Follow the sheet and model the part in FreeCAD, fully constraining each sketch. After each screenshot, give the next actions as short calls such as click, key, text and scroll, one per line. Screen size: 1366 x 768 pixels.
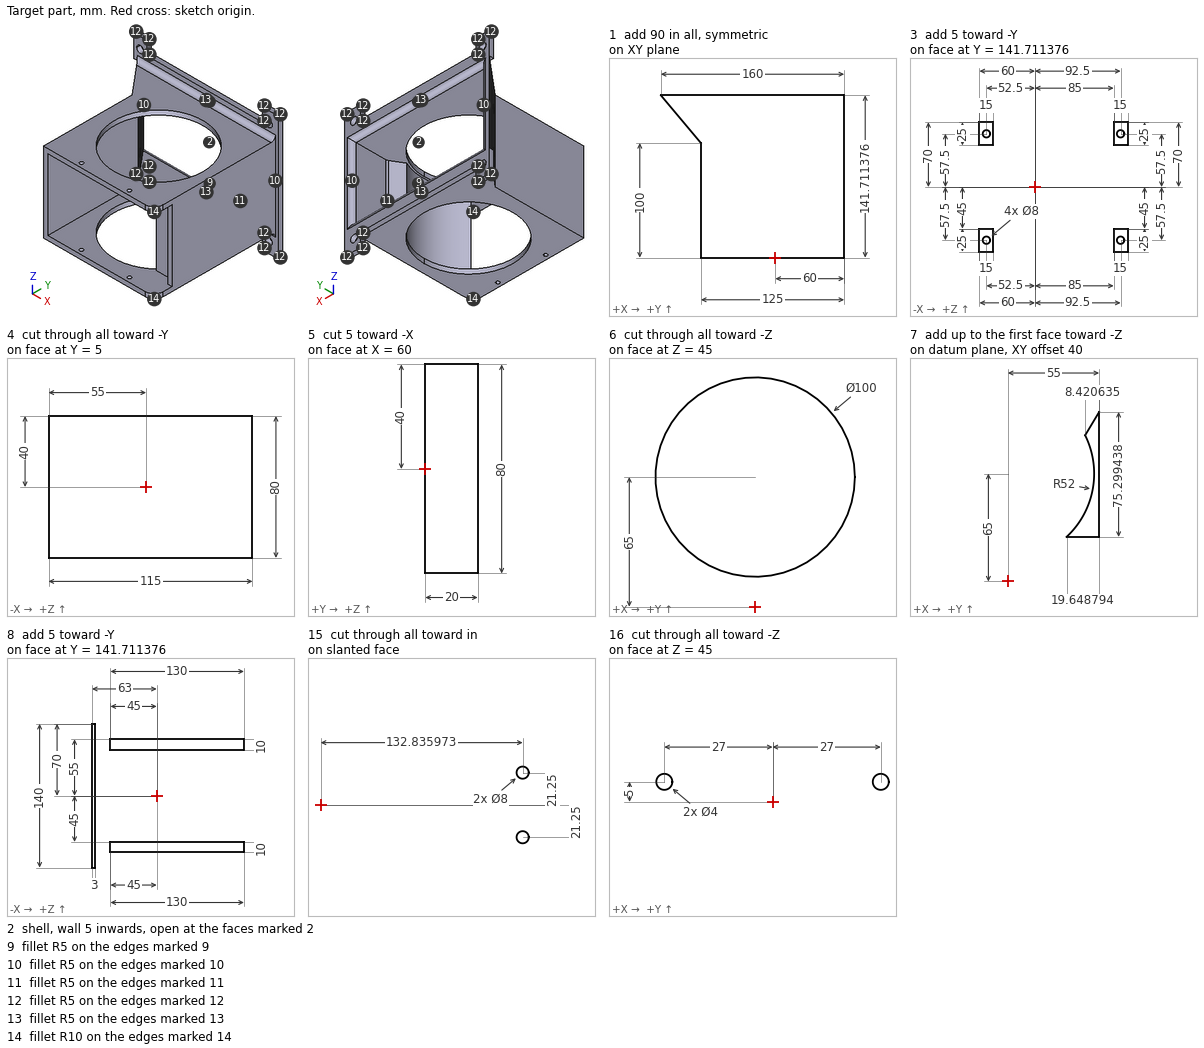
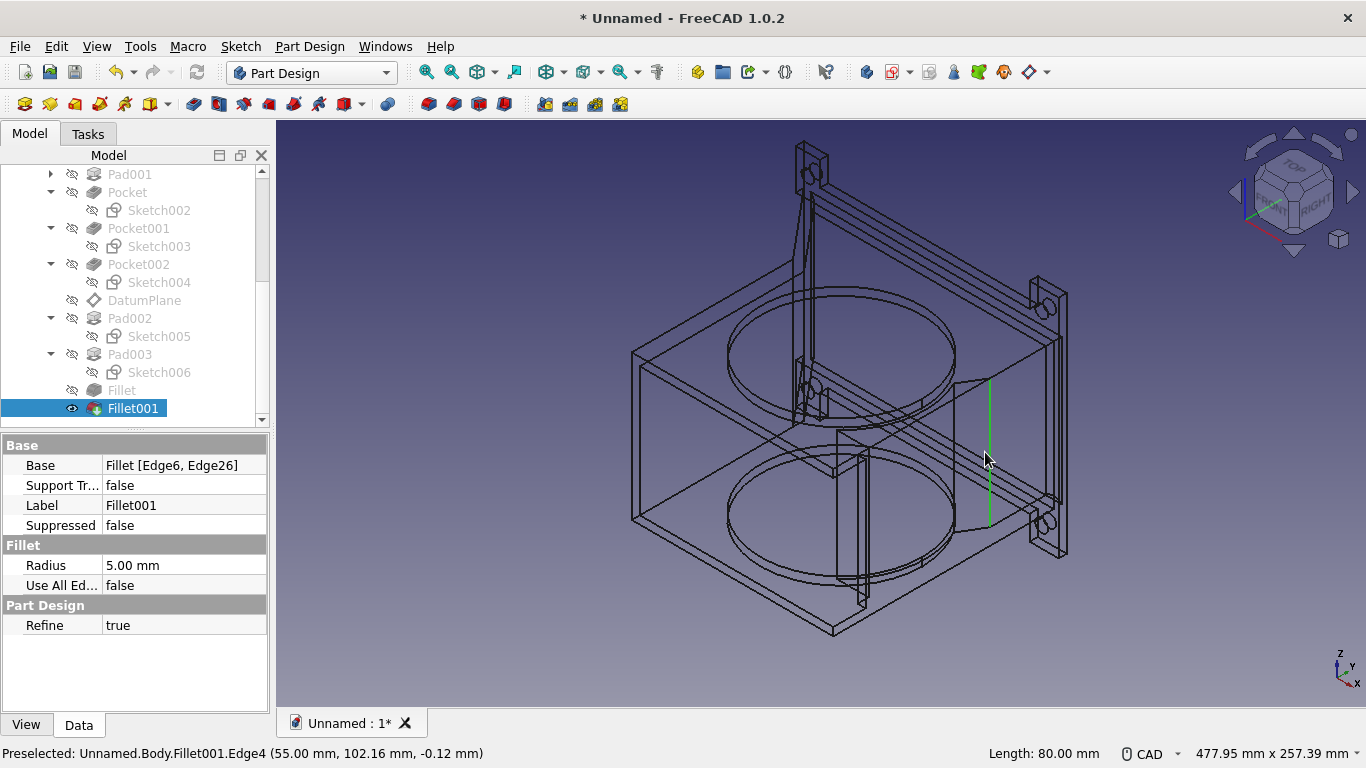
key(v)
key(1)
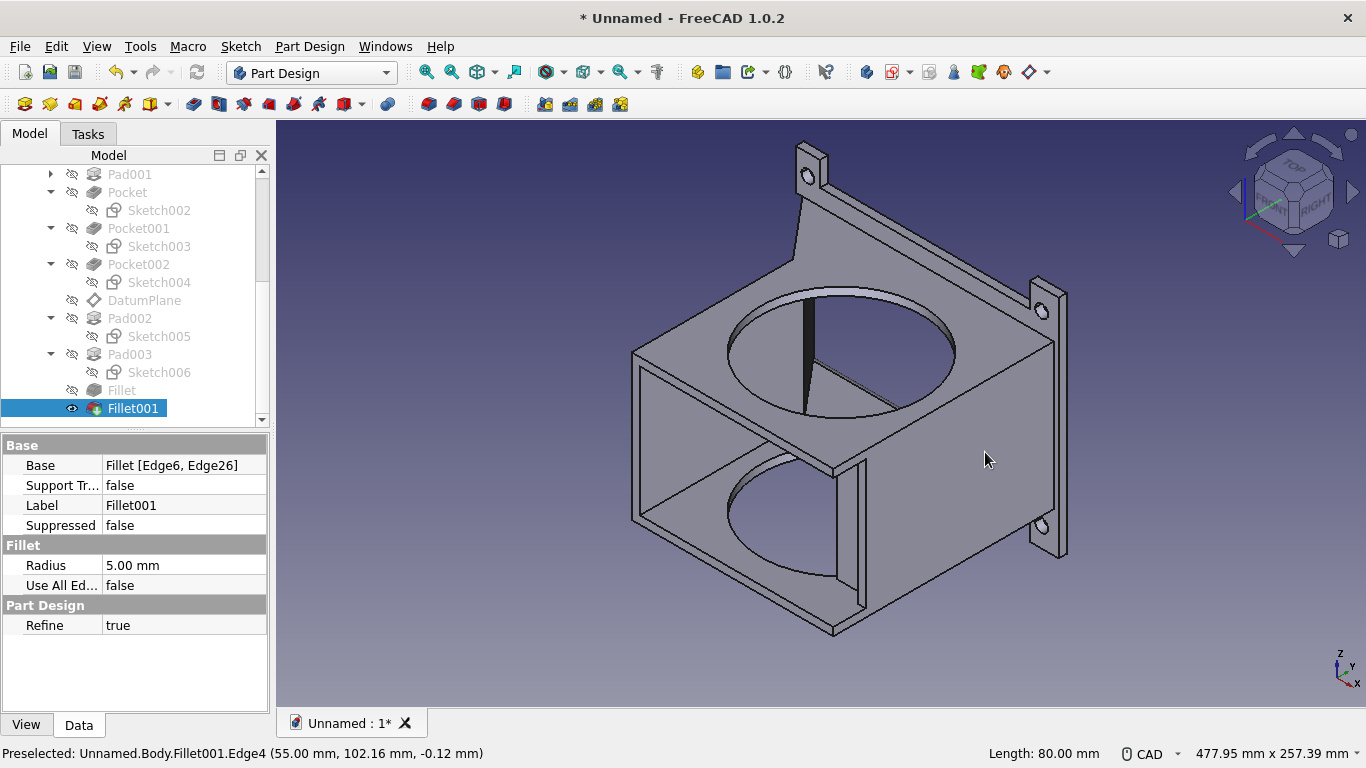
click(429, 104)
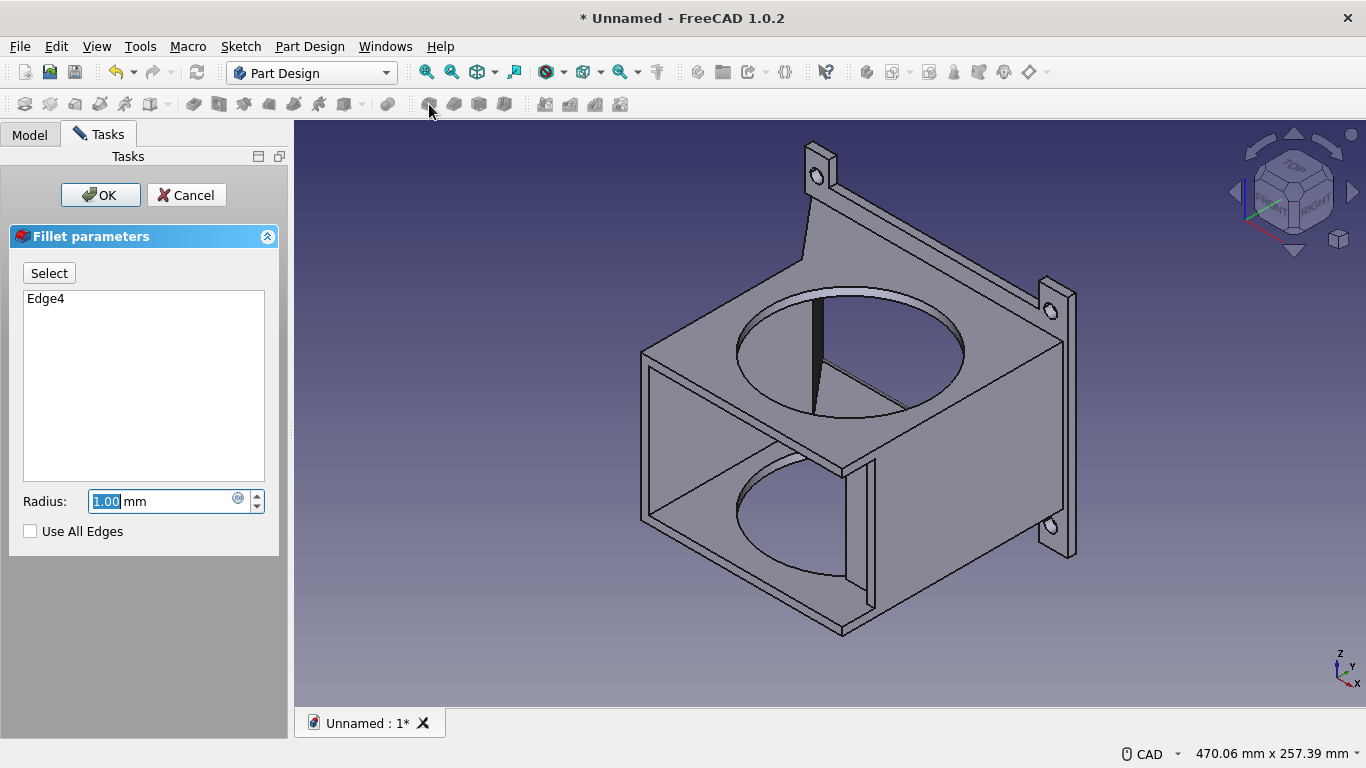
text(5)
key(Tab)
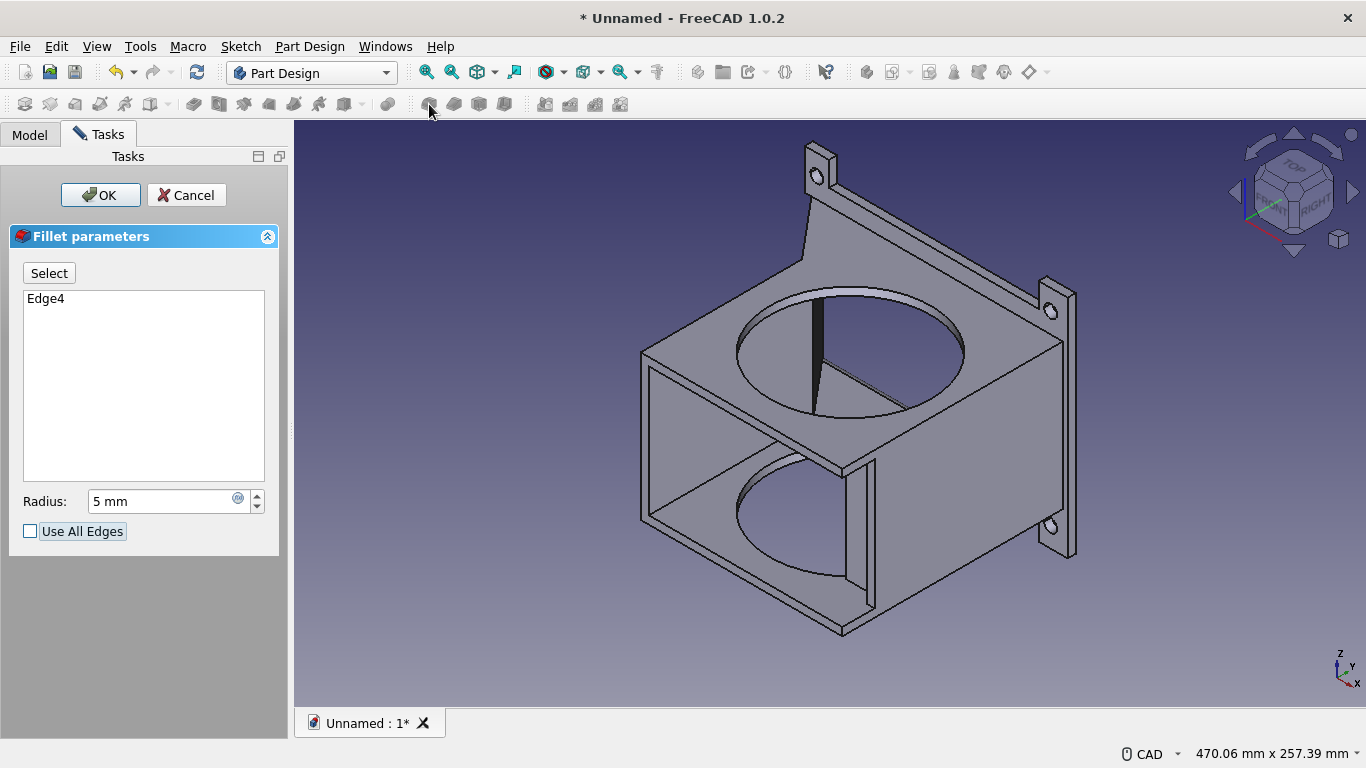
click(101, 195)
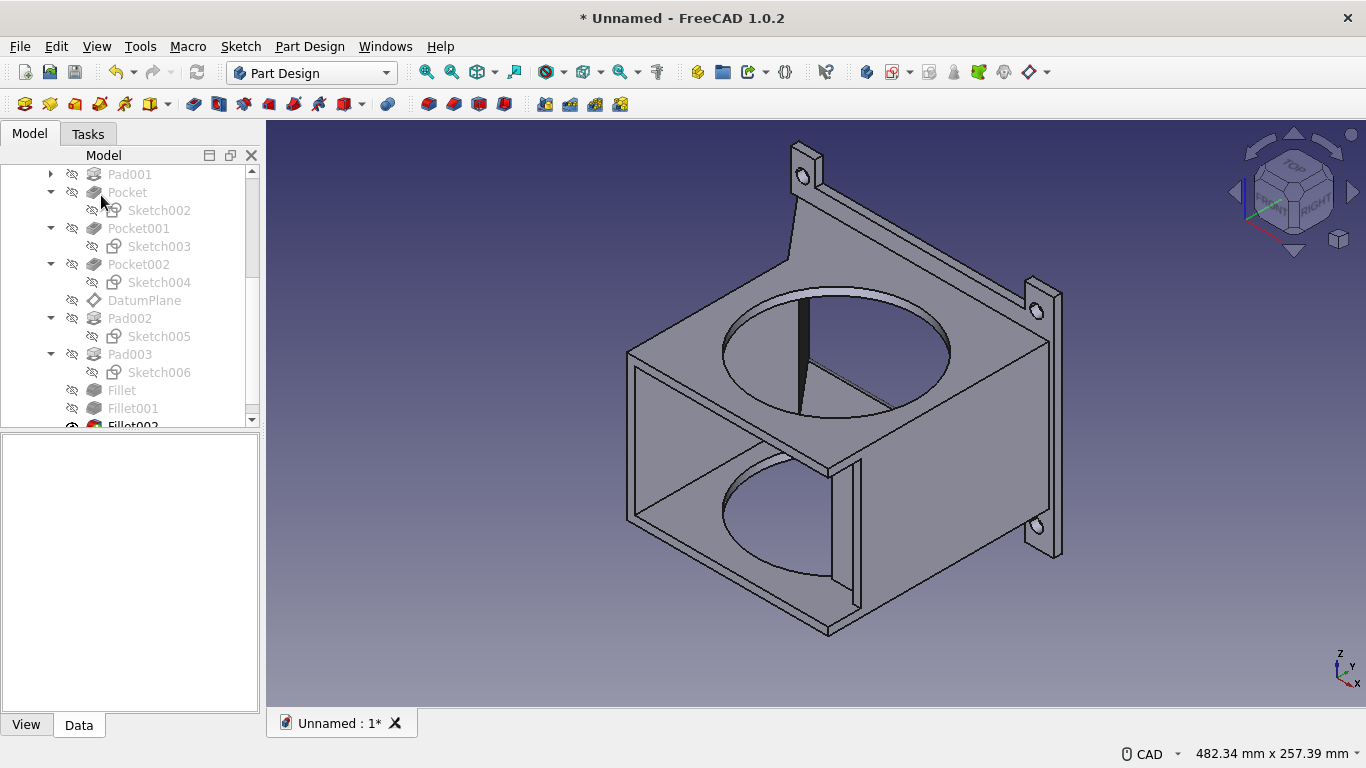
click(1059, 293)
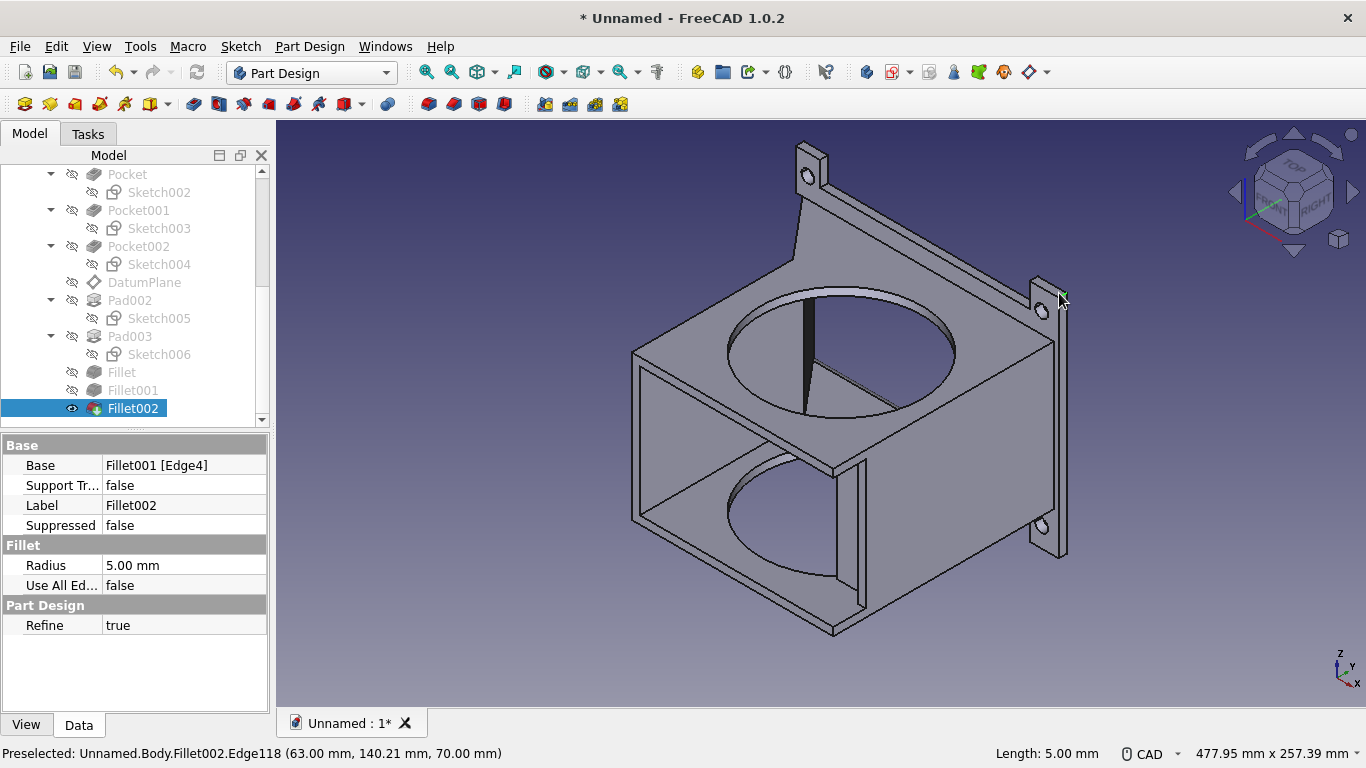
click(826, 156, ctrl)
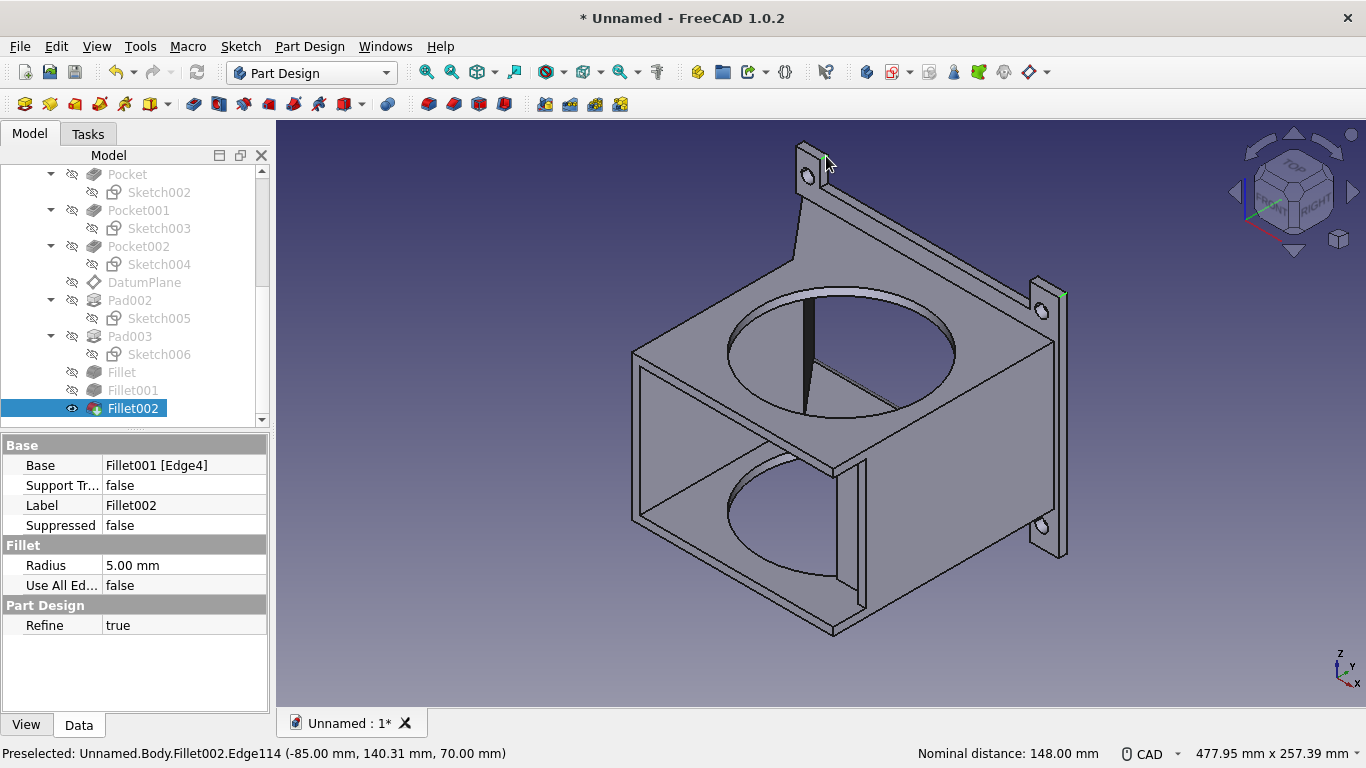
scroll(1034, 510, up, 7)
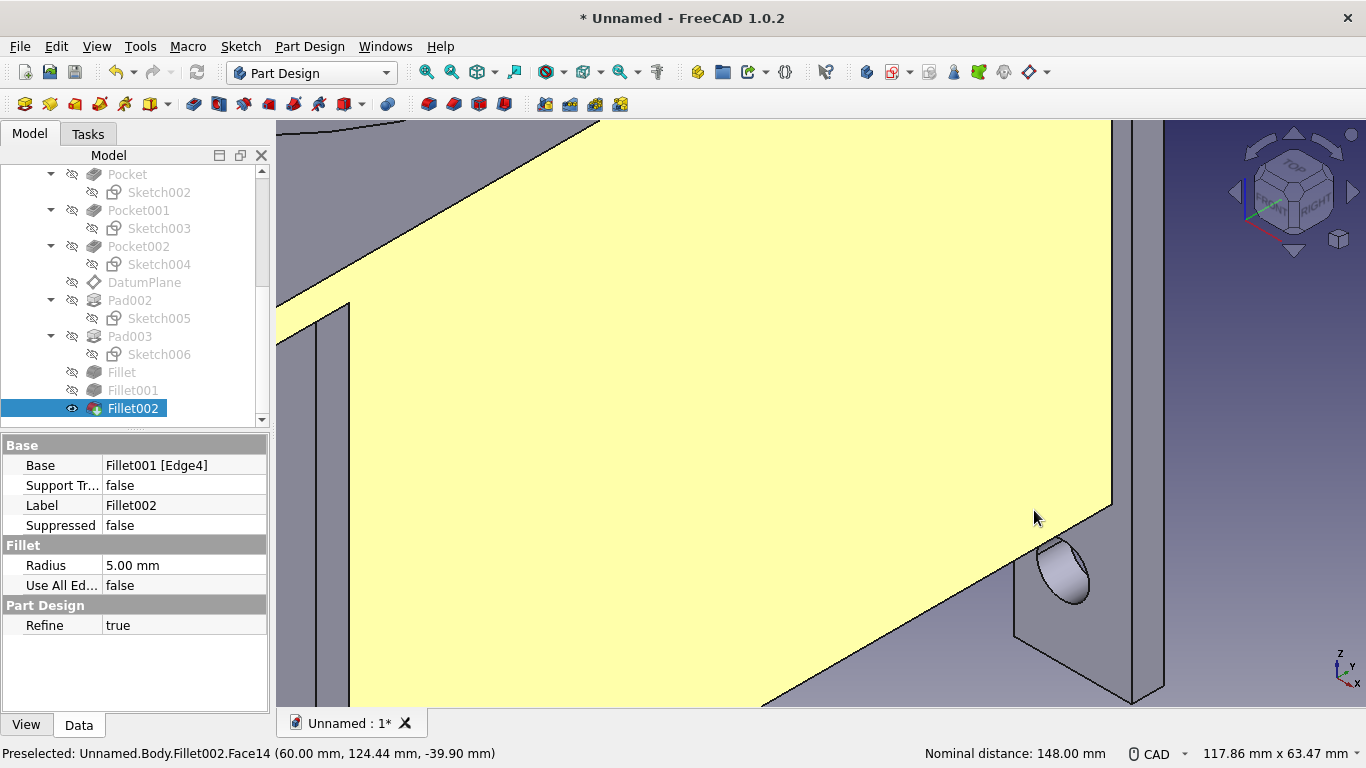
click(427, 72)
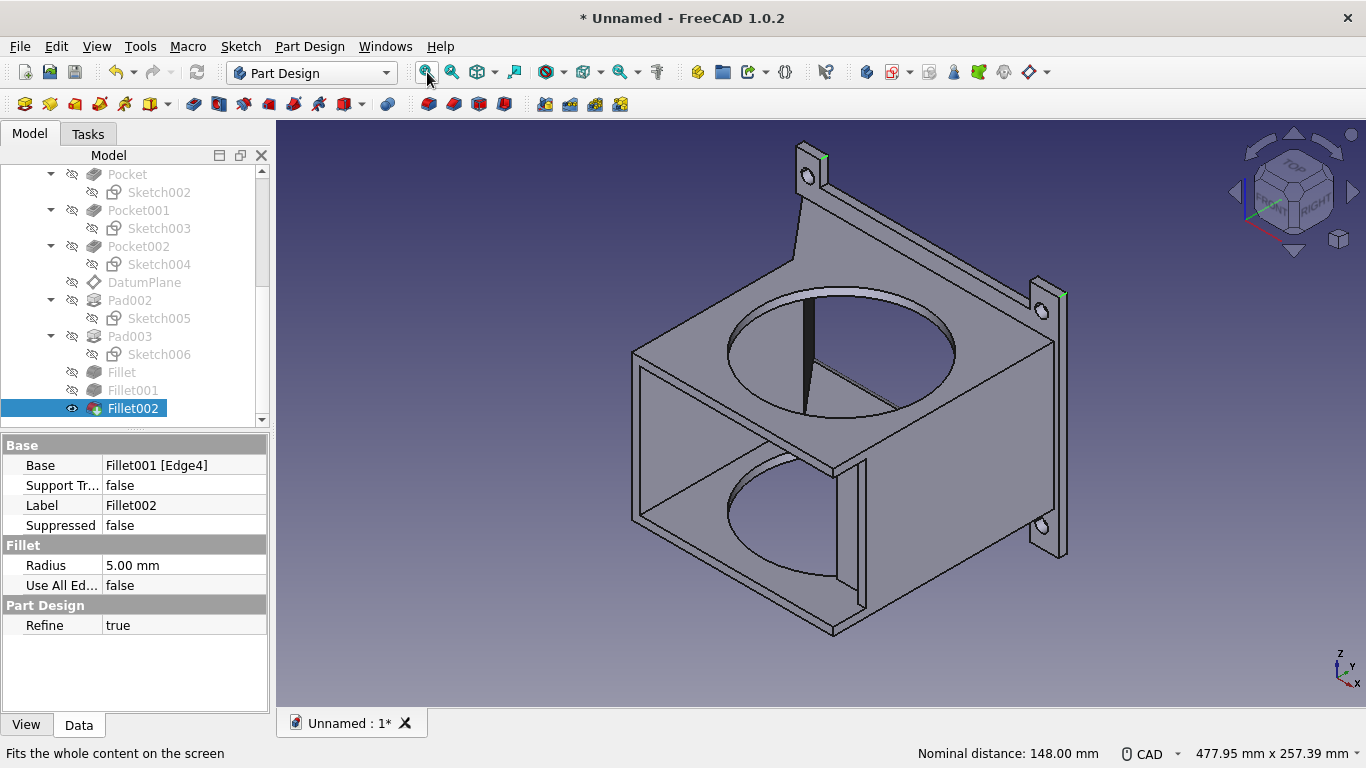
key(2)